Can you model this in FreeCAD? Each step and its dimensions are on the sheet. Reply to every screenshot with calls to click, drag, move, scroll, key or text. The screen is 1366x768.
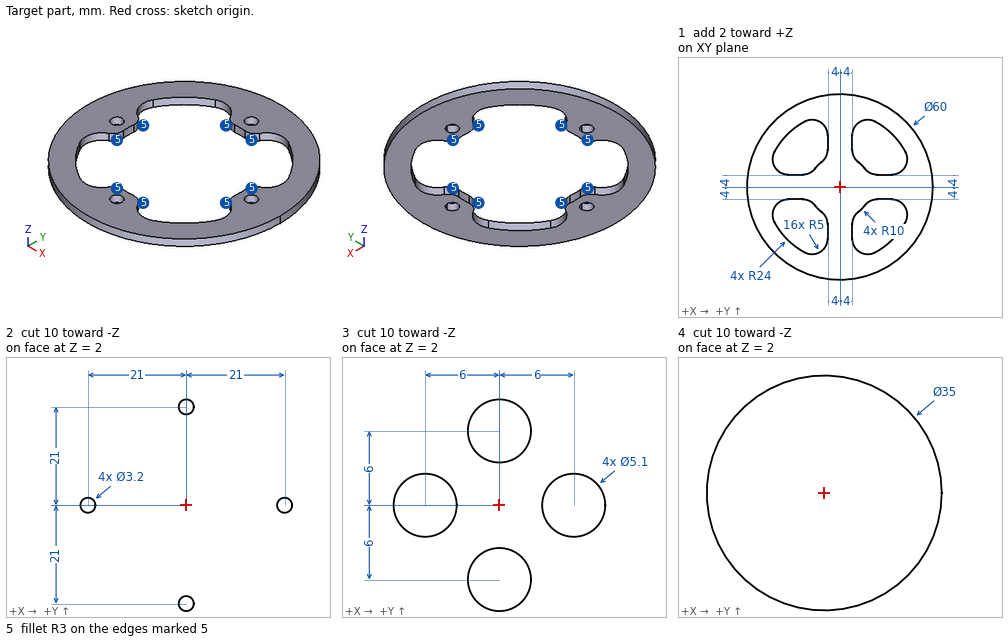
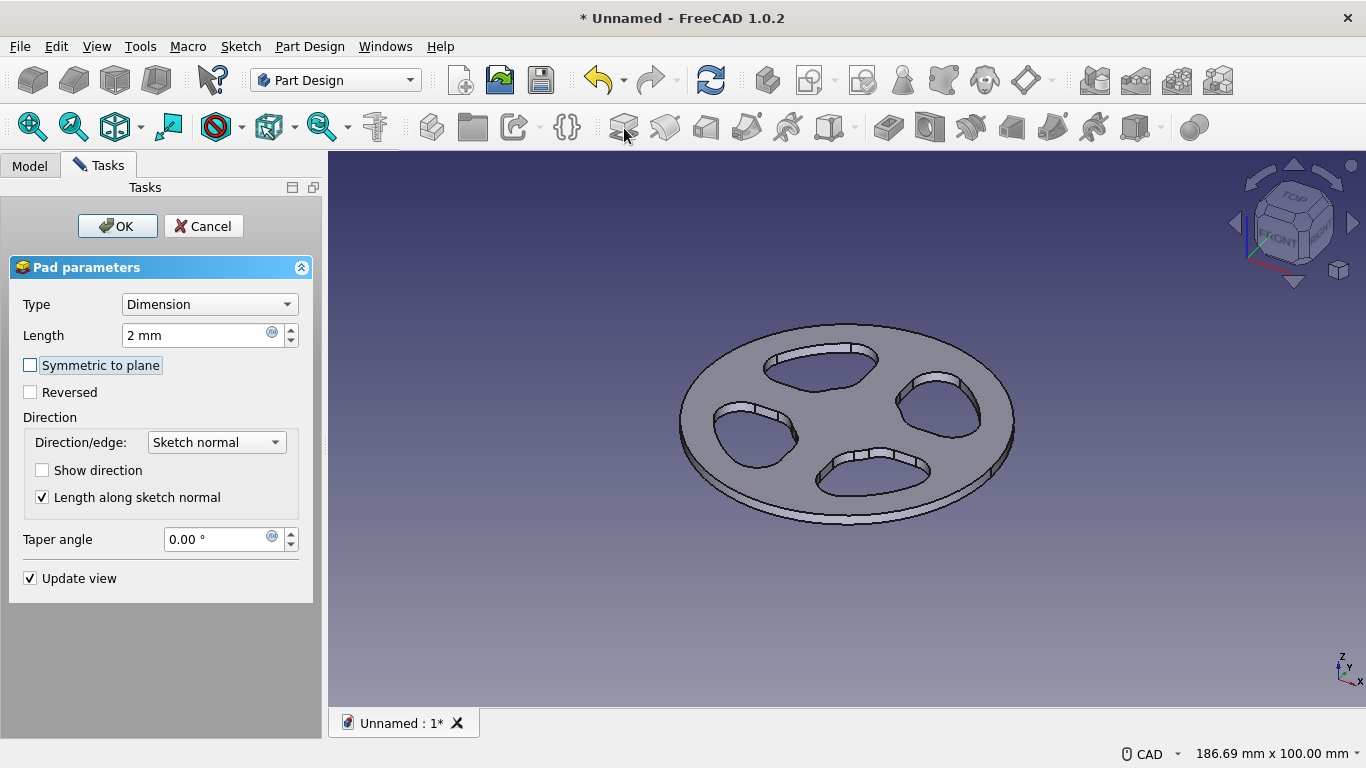
click(118, 226)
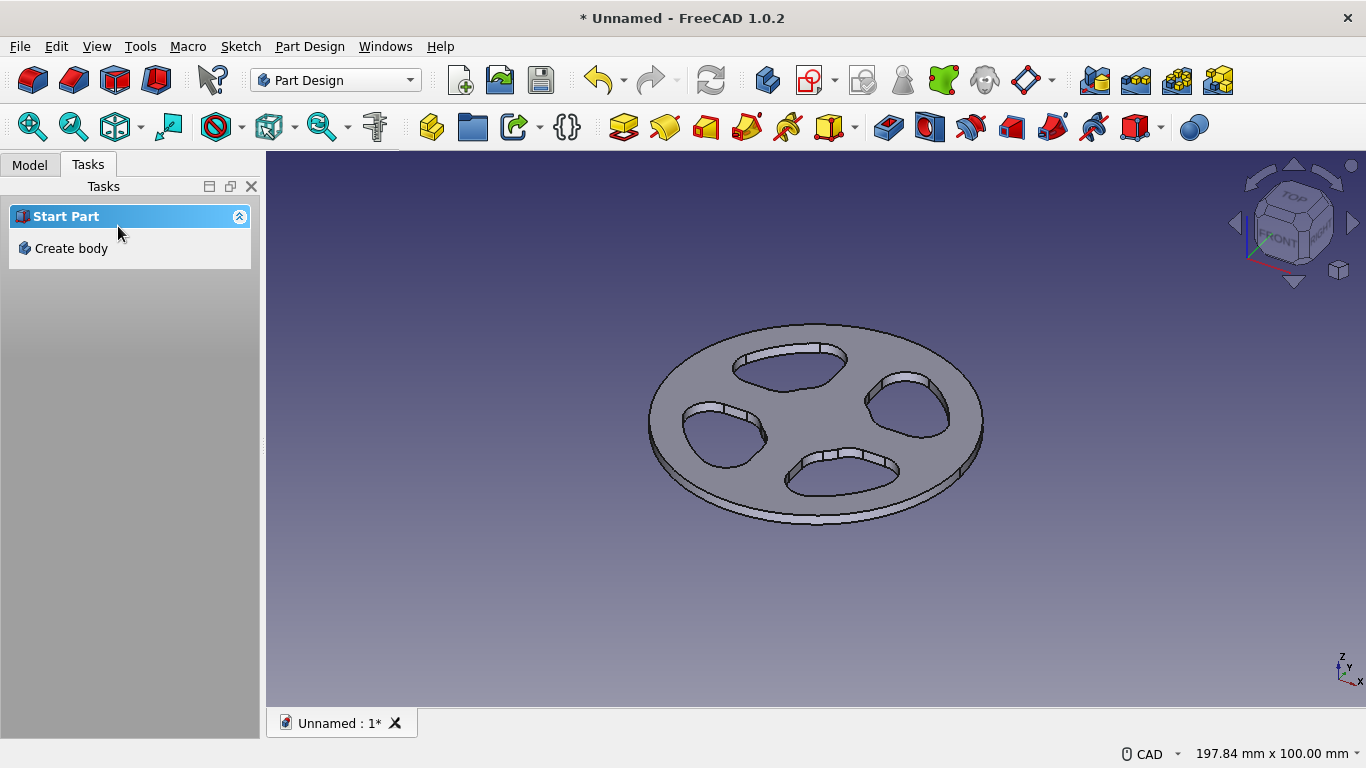
click(816, 419)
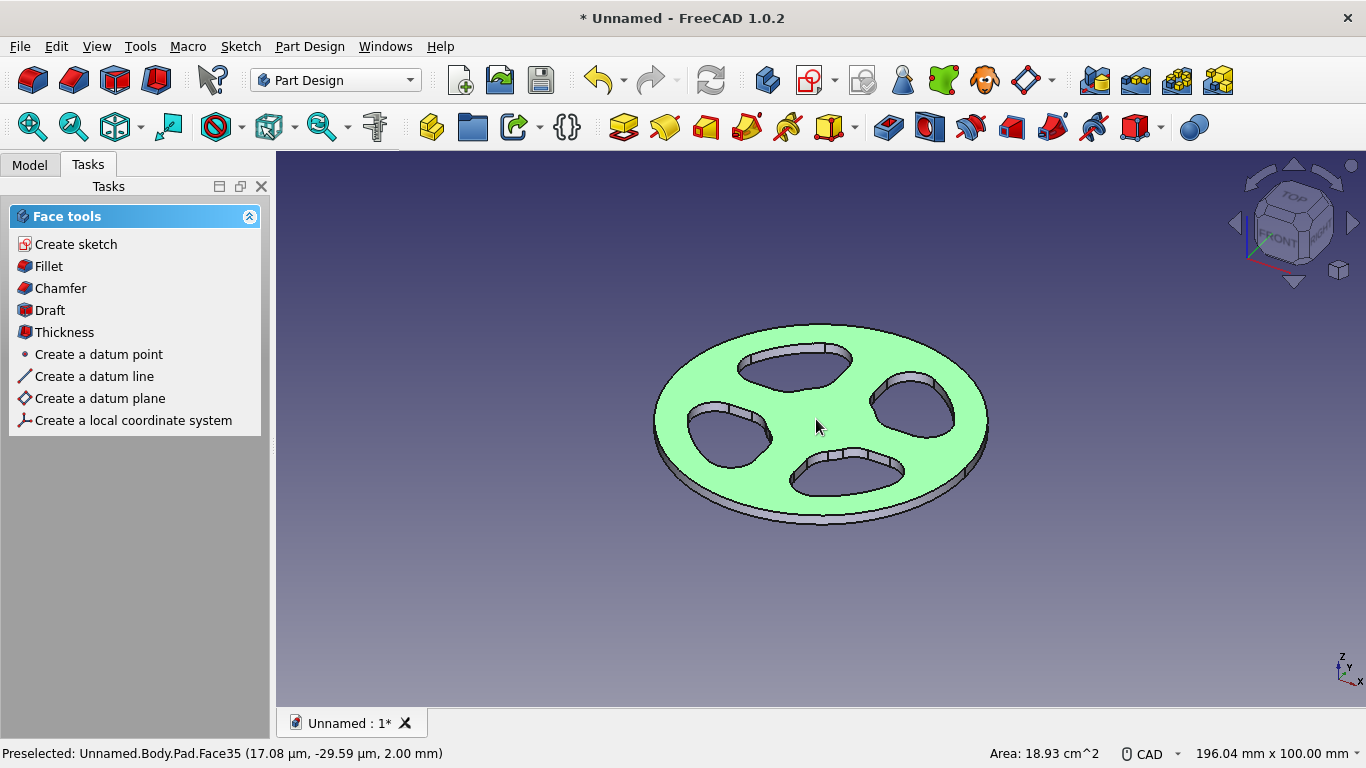
click(808, 80)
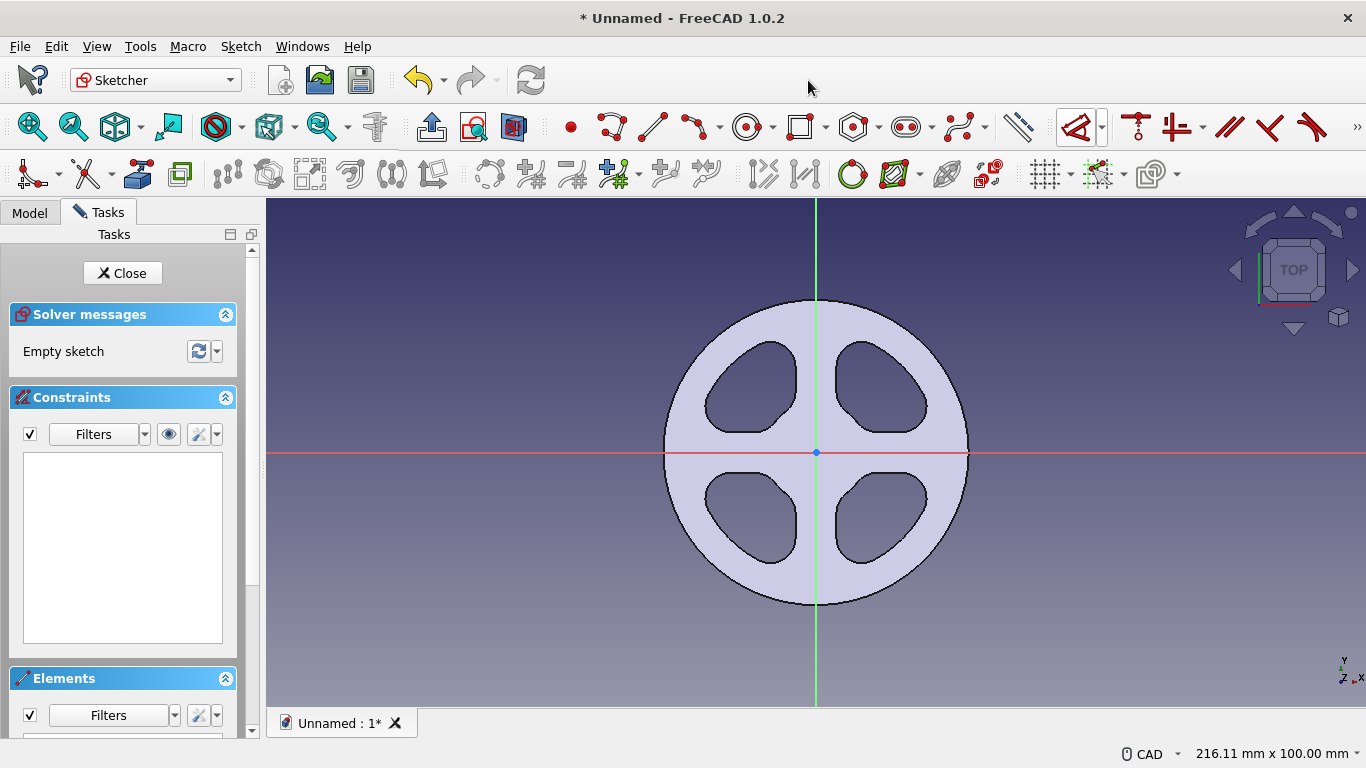
scroll(955, 453, up, 2)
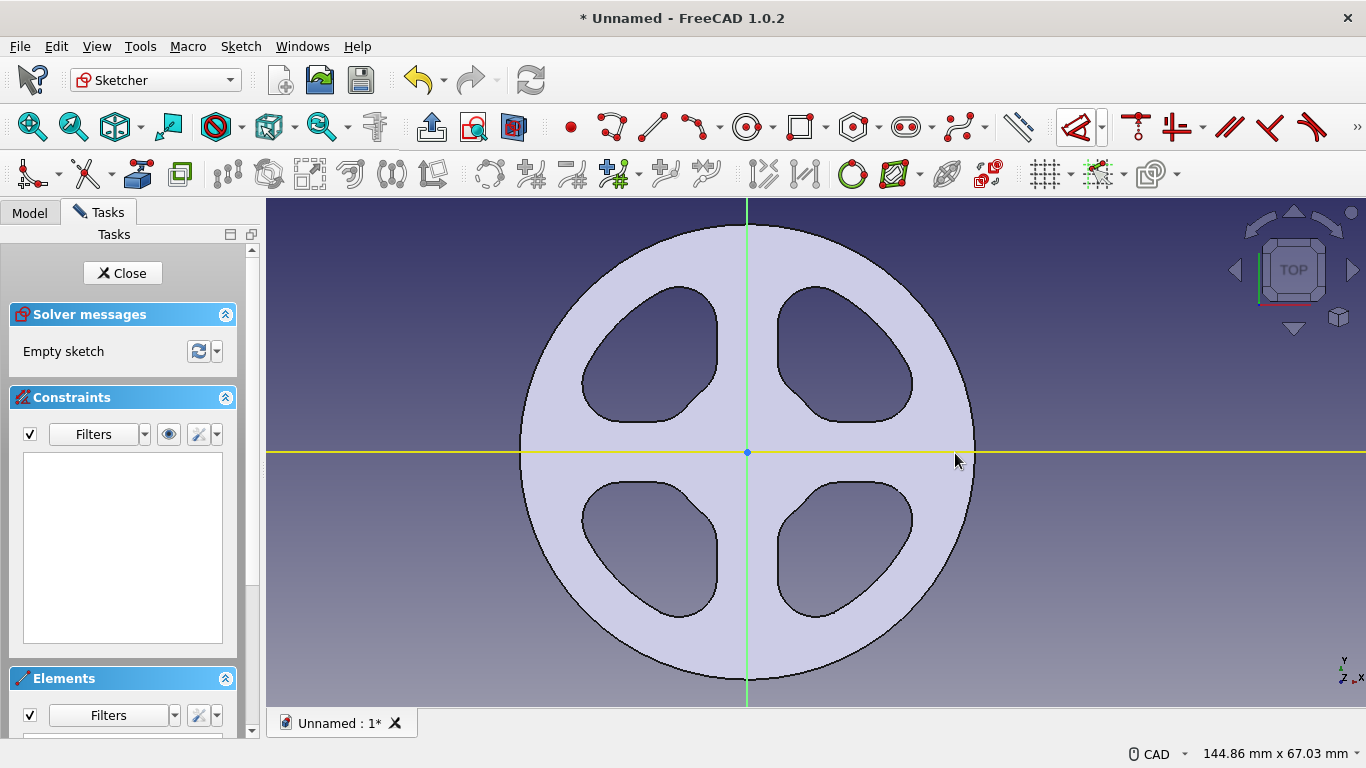
key(g)
key(c)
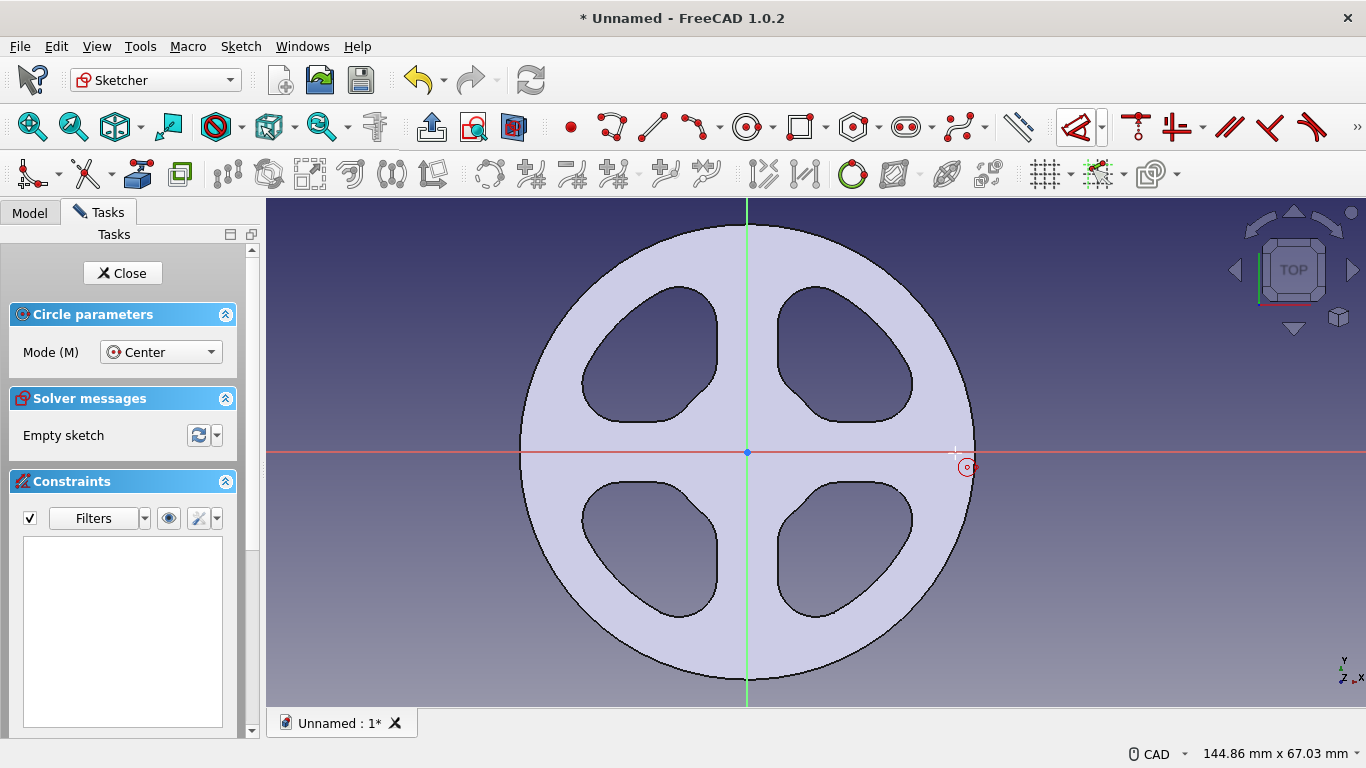
scroll(588, 452, up, 4)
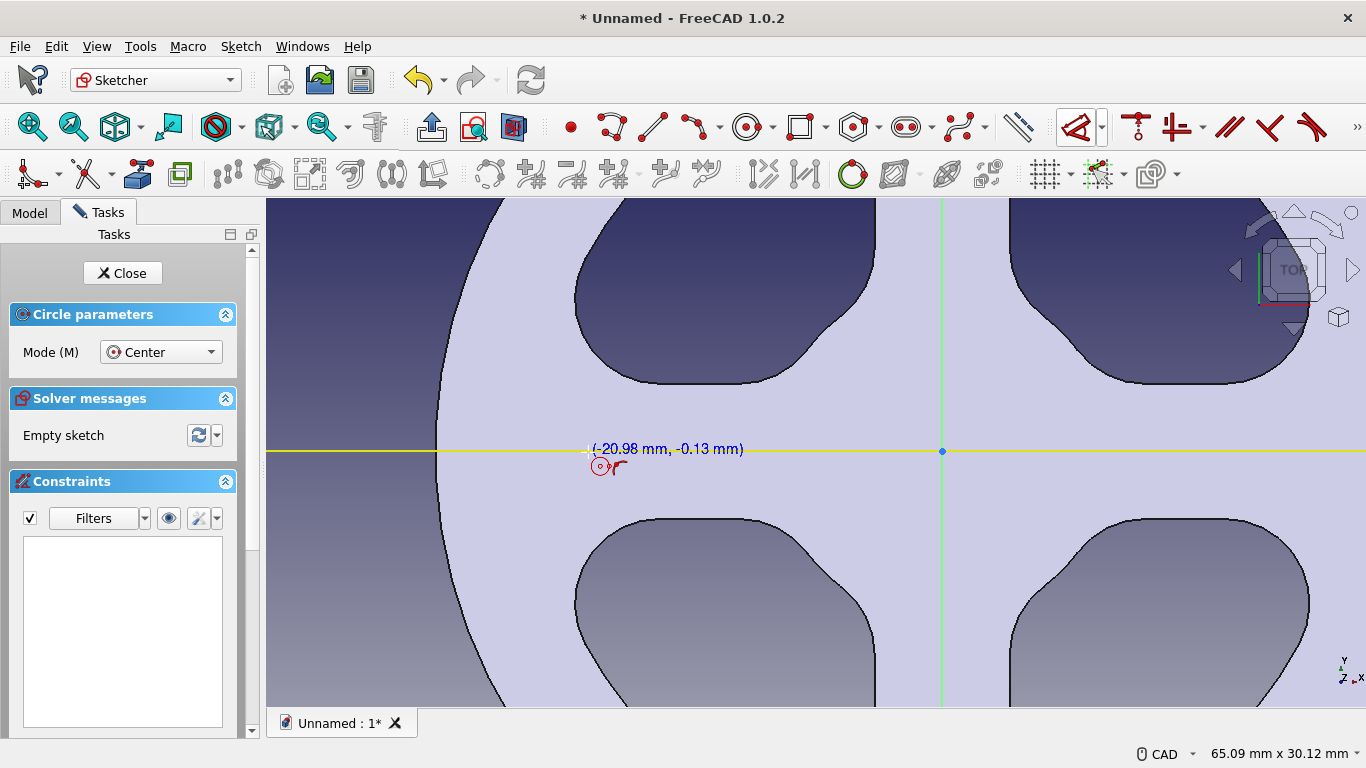
click(587, 451)
click(606, 432)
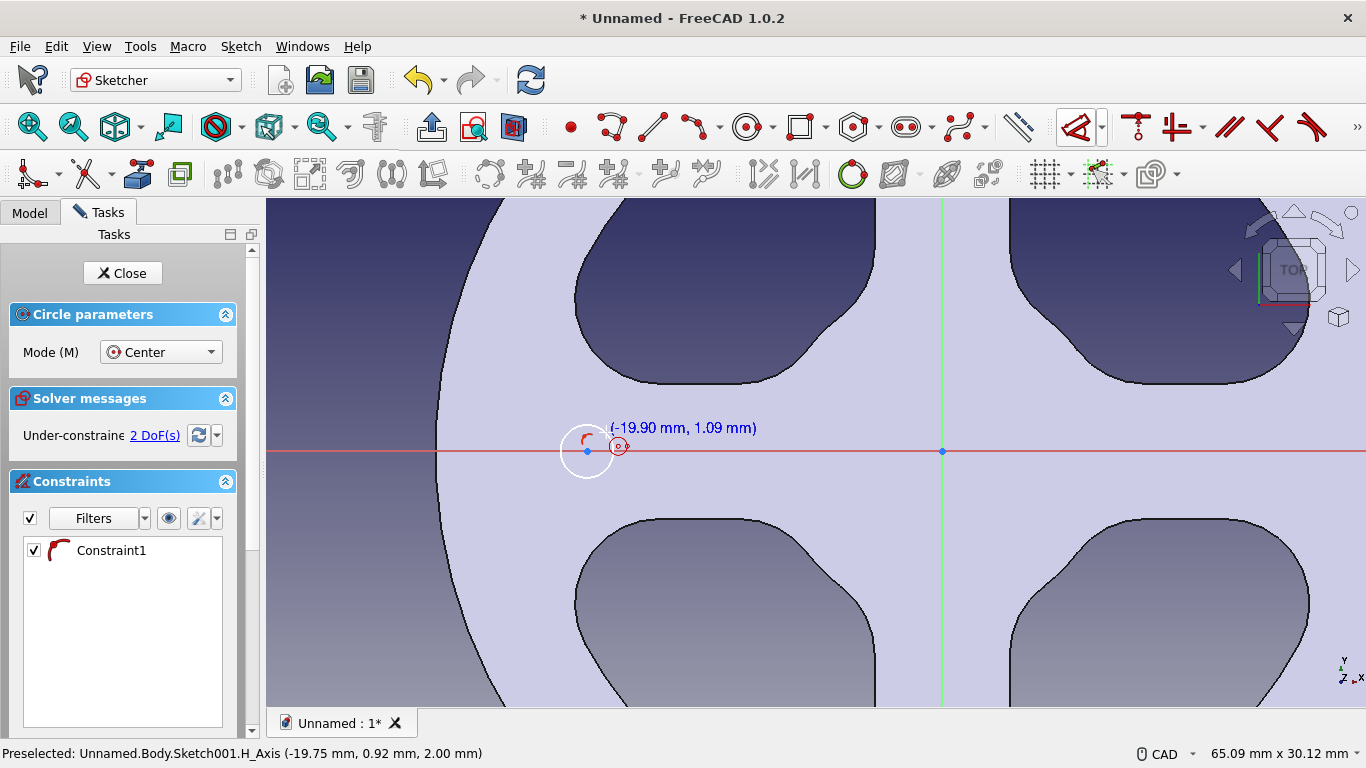
scroll(589, 453, down, 4)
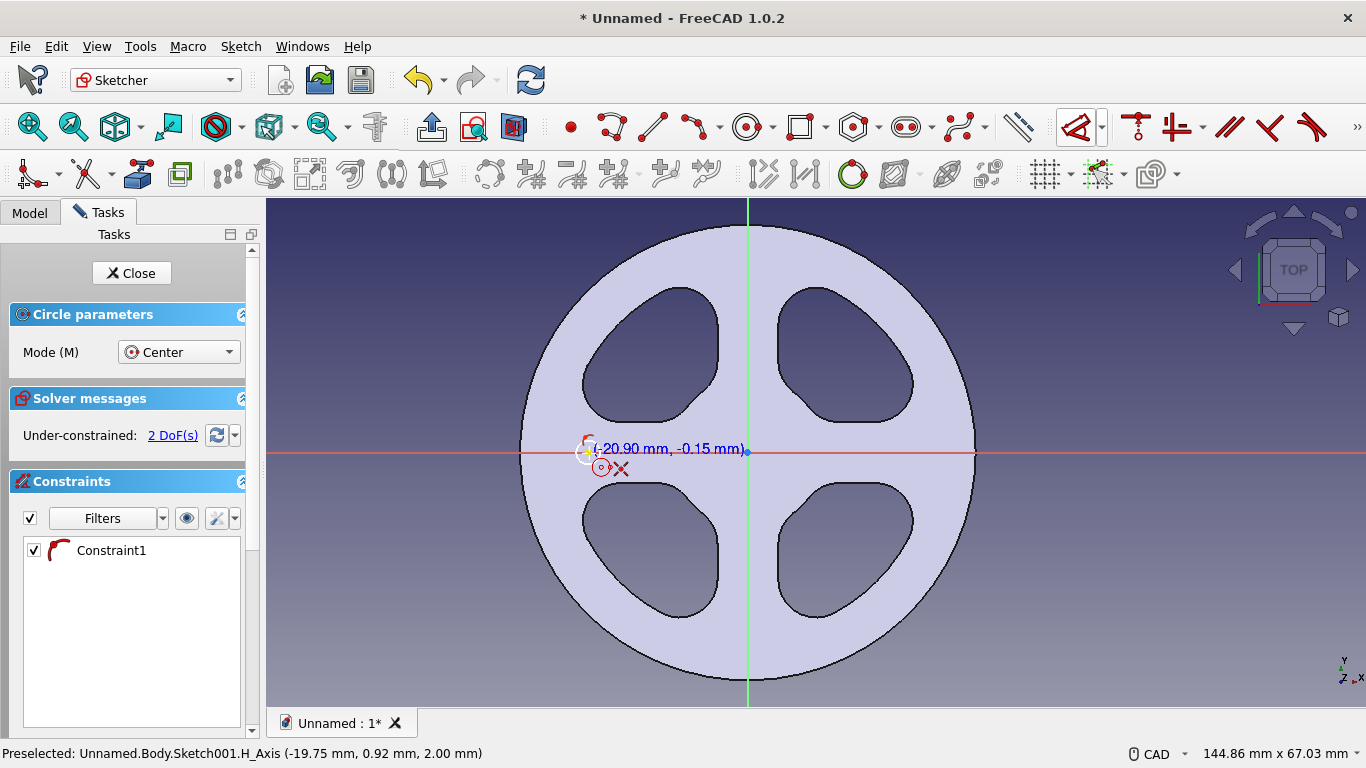
scroll(748, 293, up, 4)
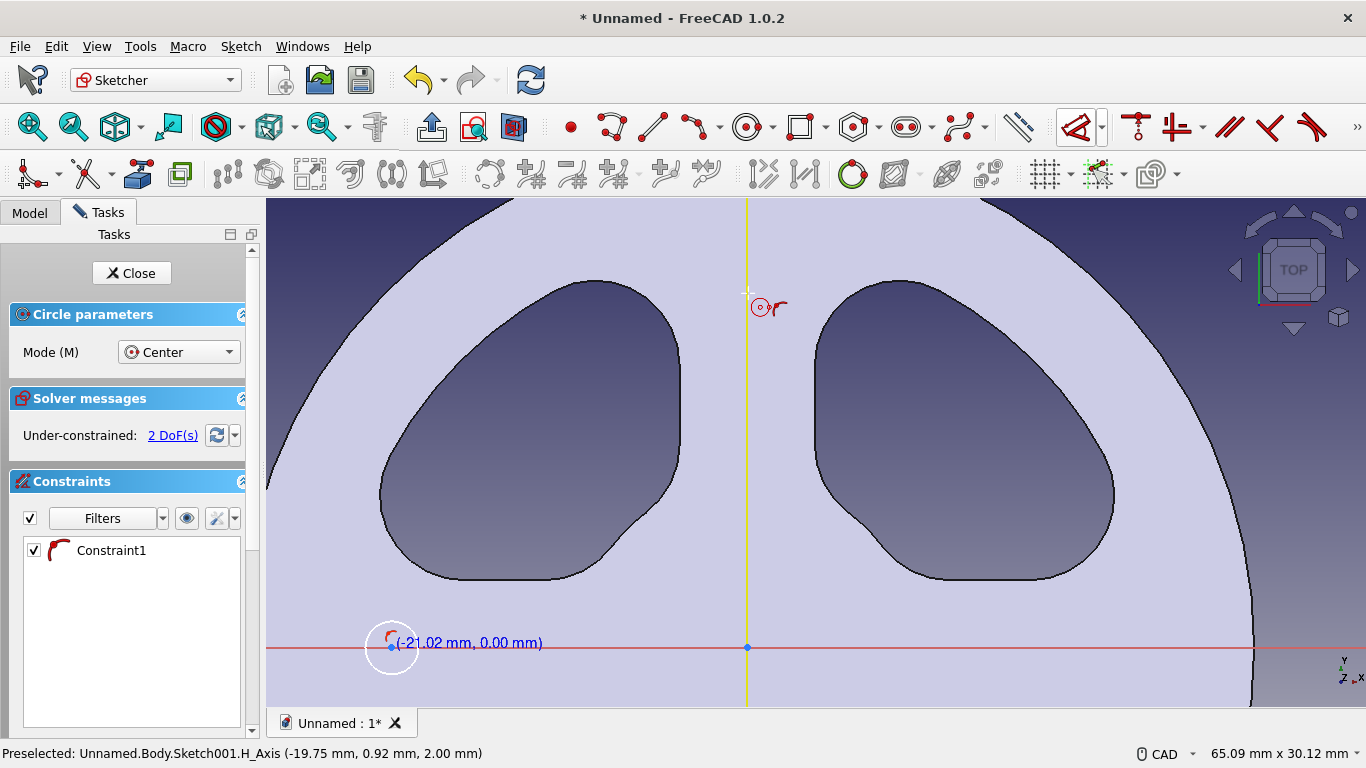
click(747, 293)
click(766, 274)